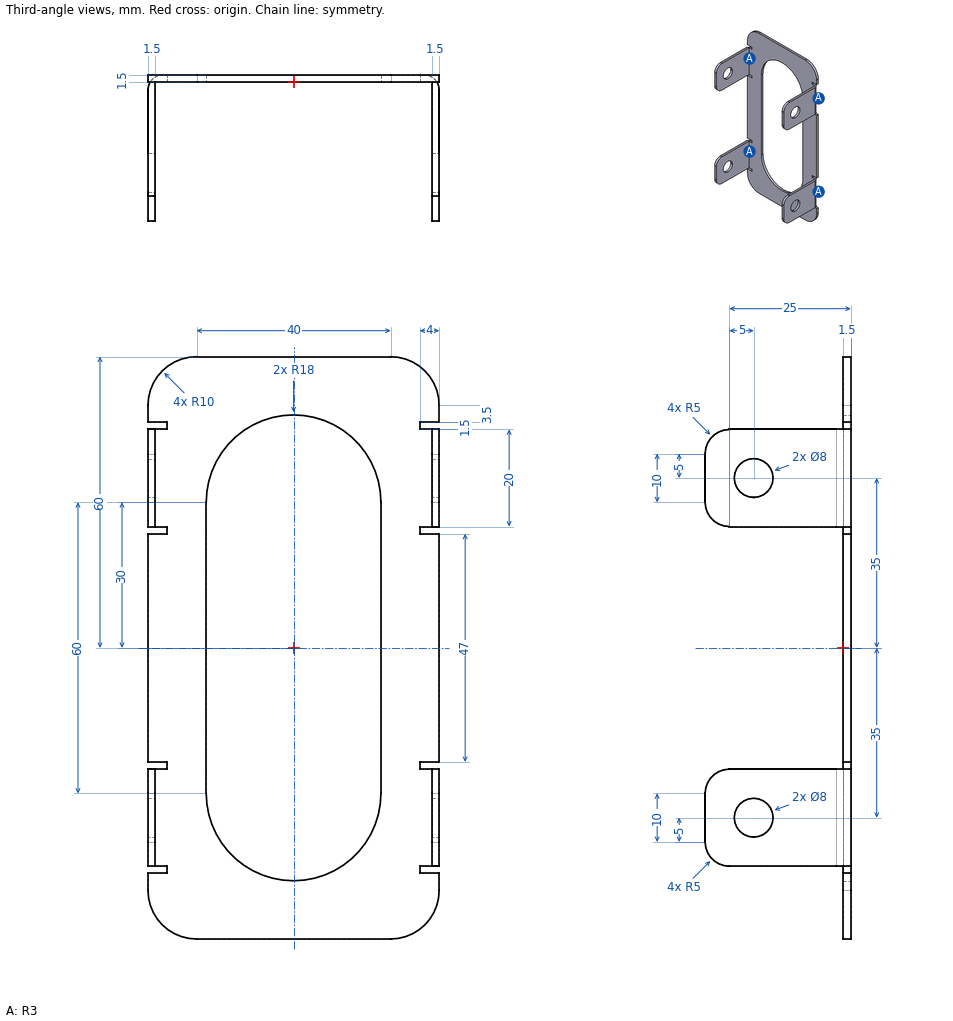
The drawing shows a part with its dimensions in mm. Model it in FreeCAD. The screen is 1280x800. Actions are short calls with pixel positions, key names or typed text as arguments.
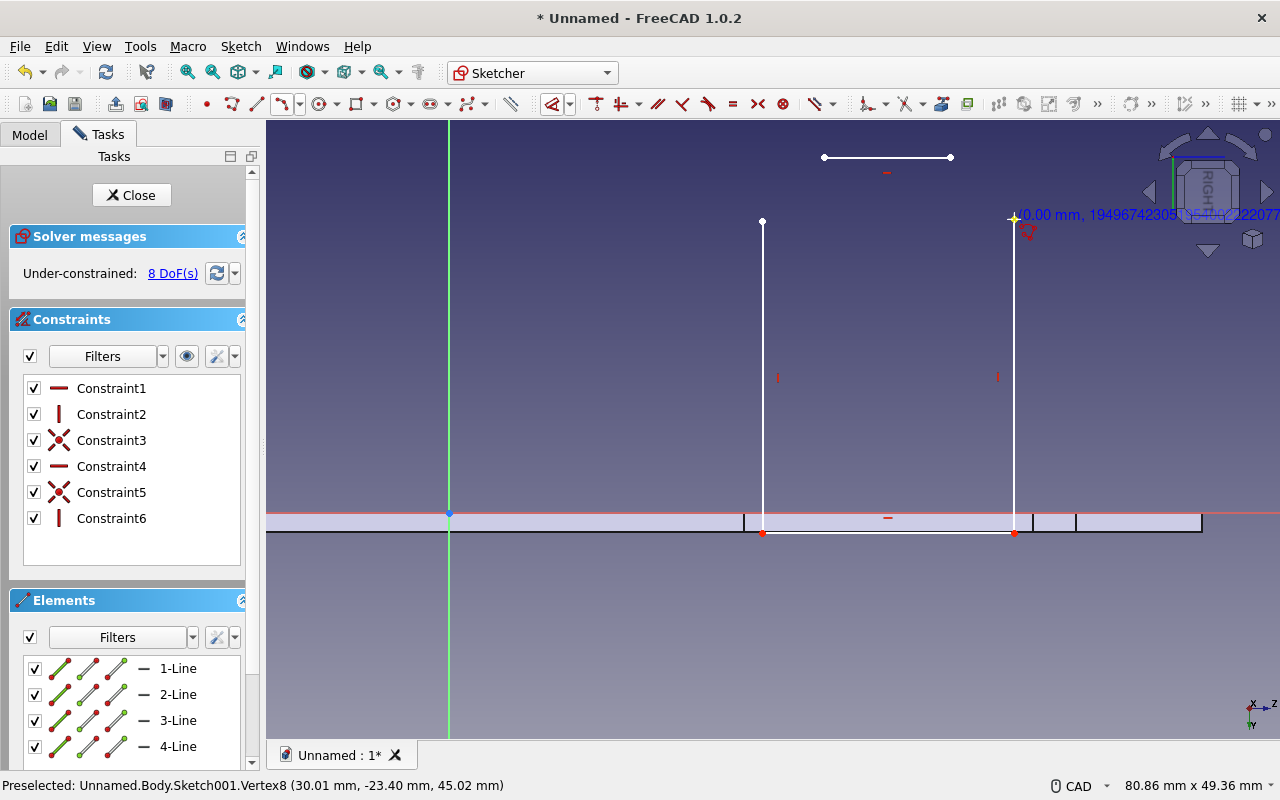
click(282, 104)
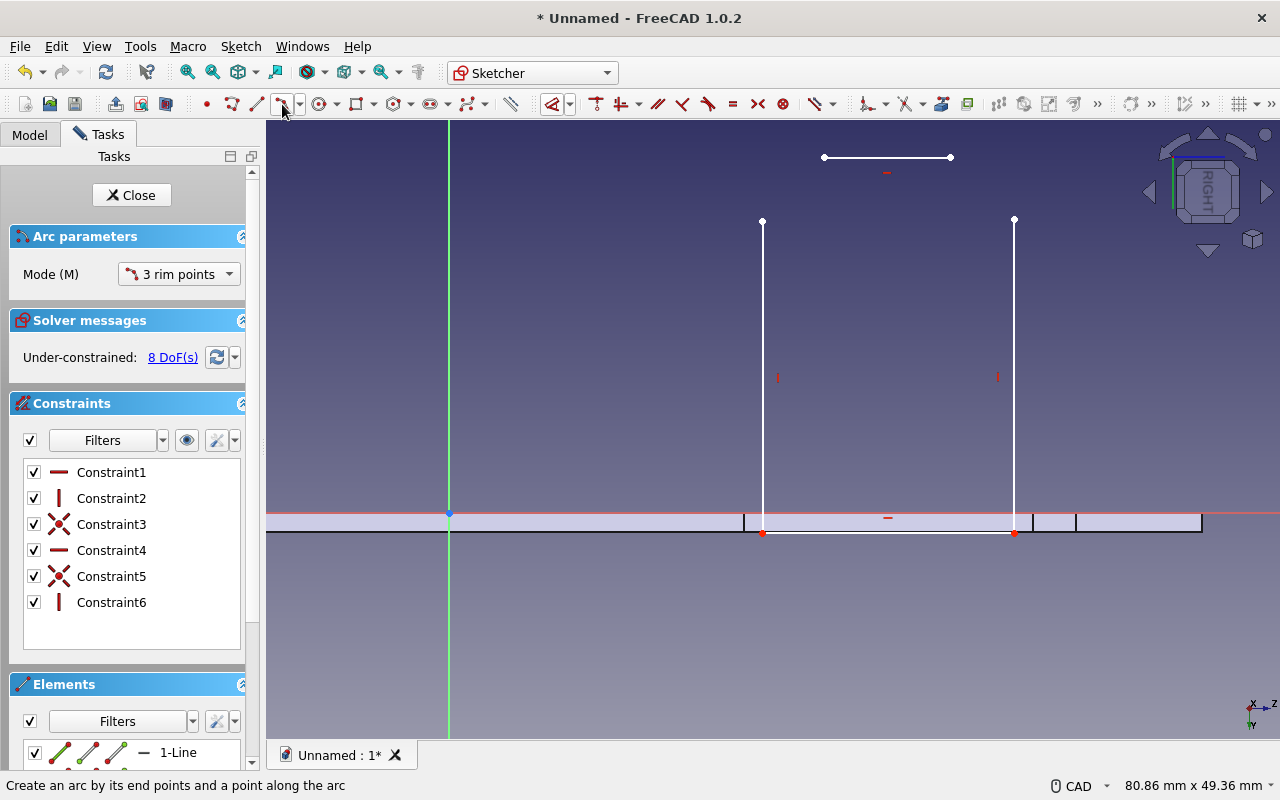
click(825, 158)
click(763, 221)
click(781, 174)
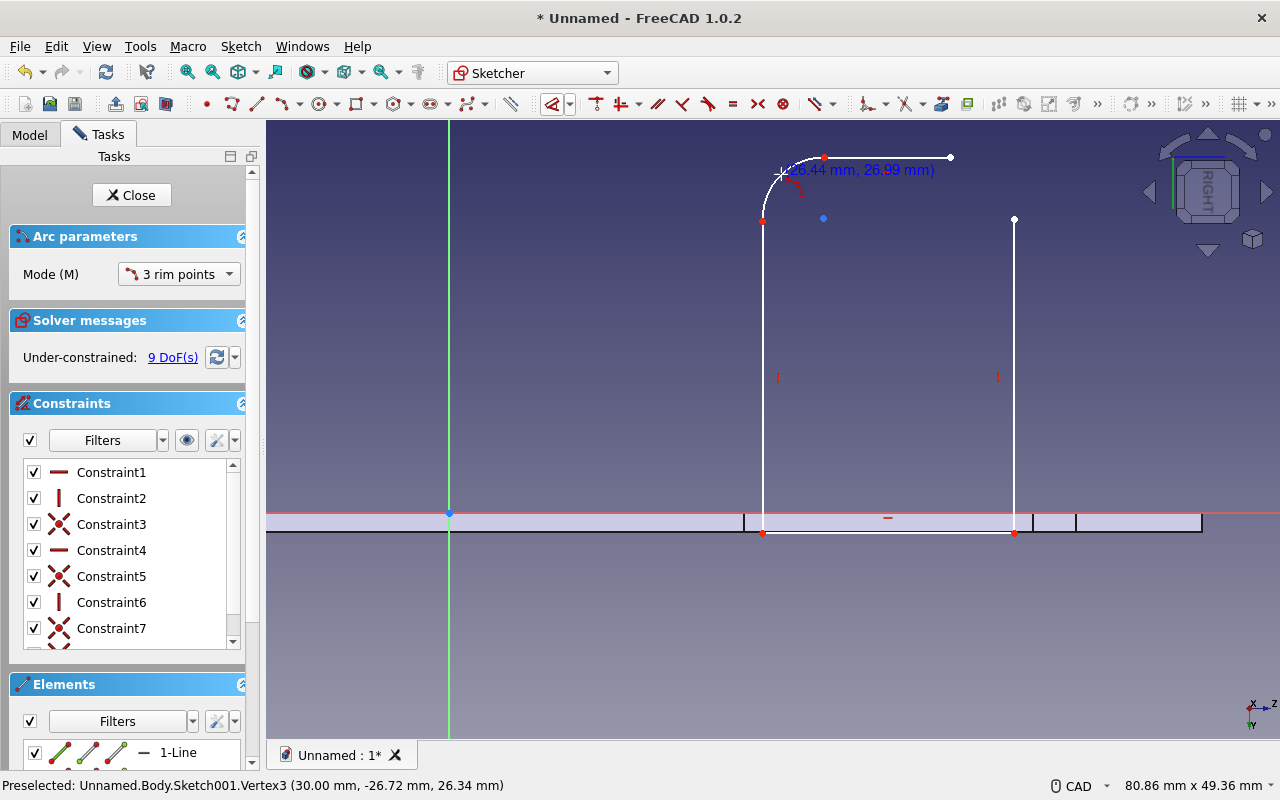
click(1014, 220)
click(951, 158)
click(995, 174)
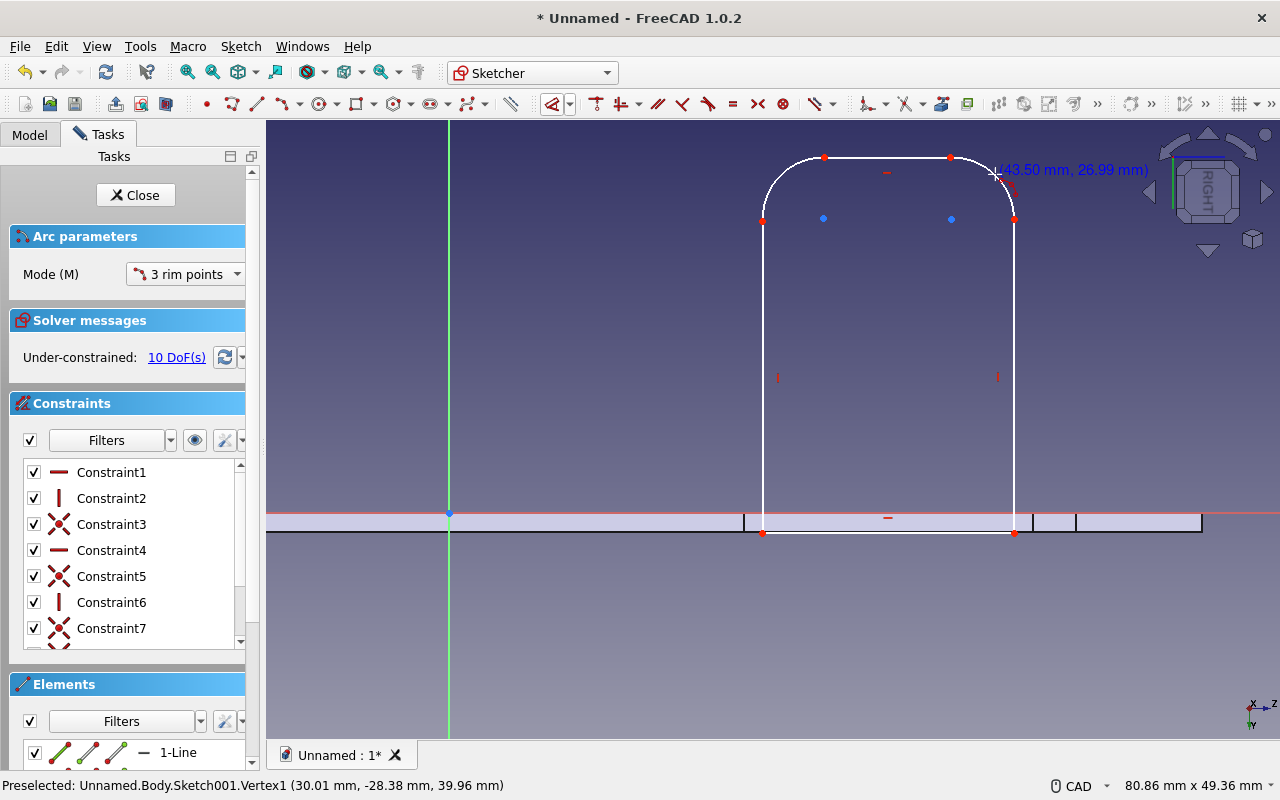
click(257, 104)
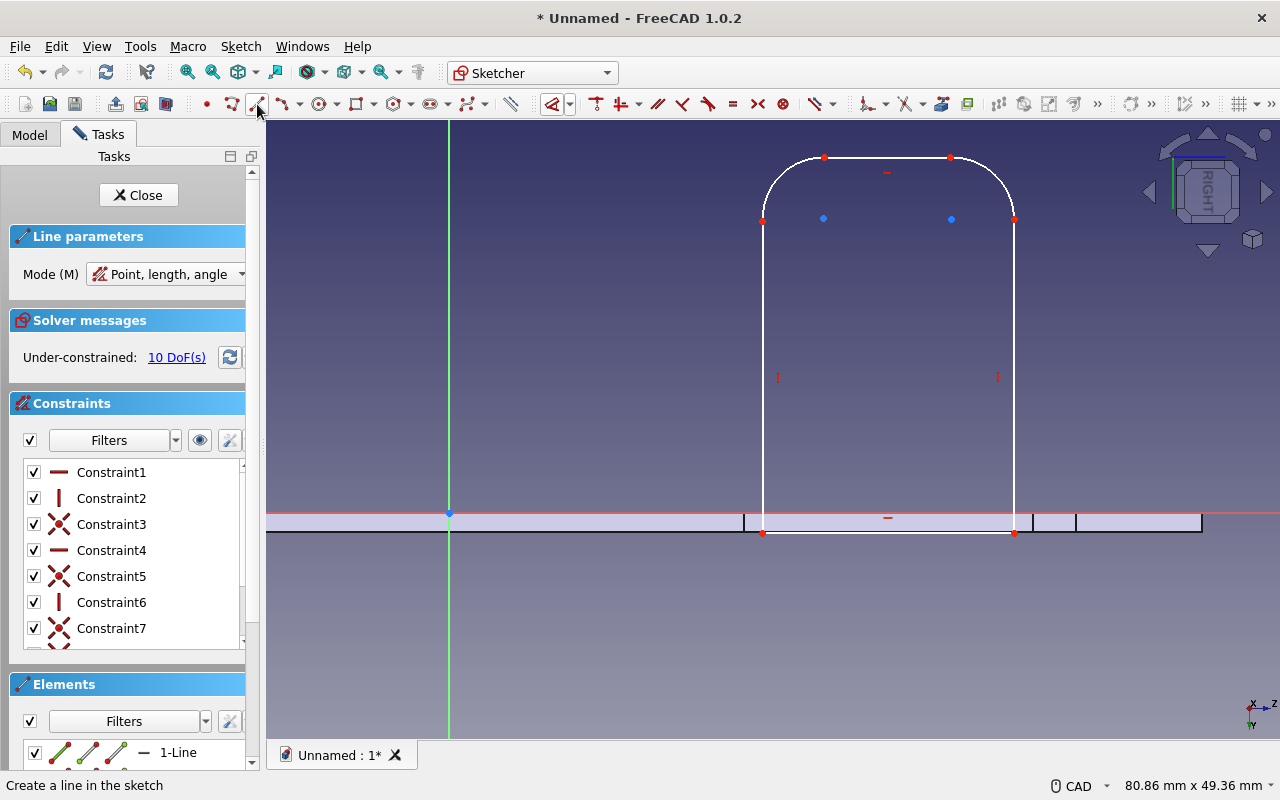
scroll(1015, 533, down, 3)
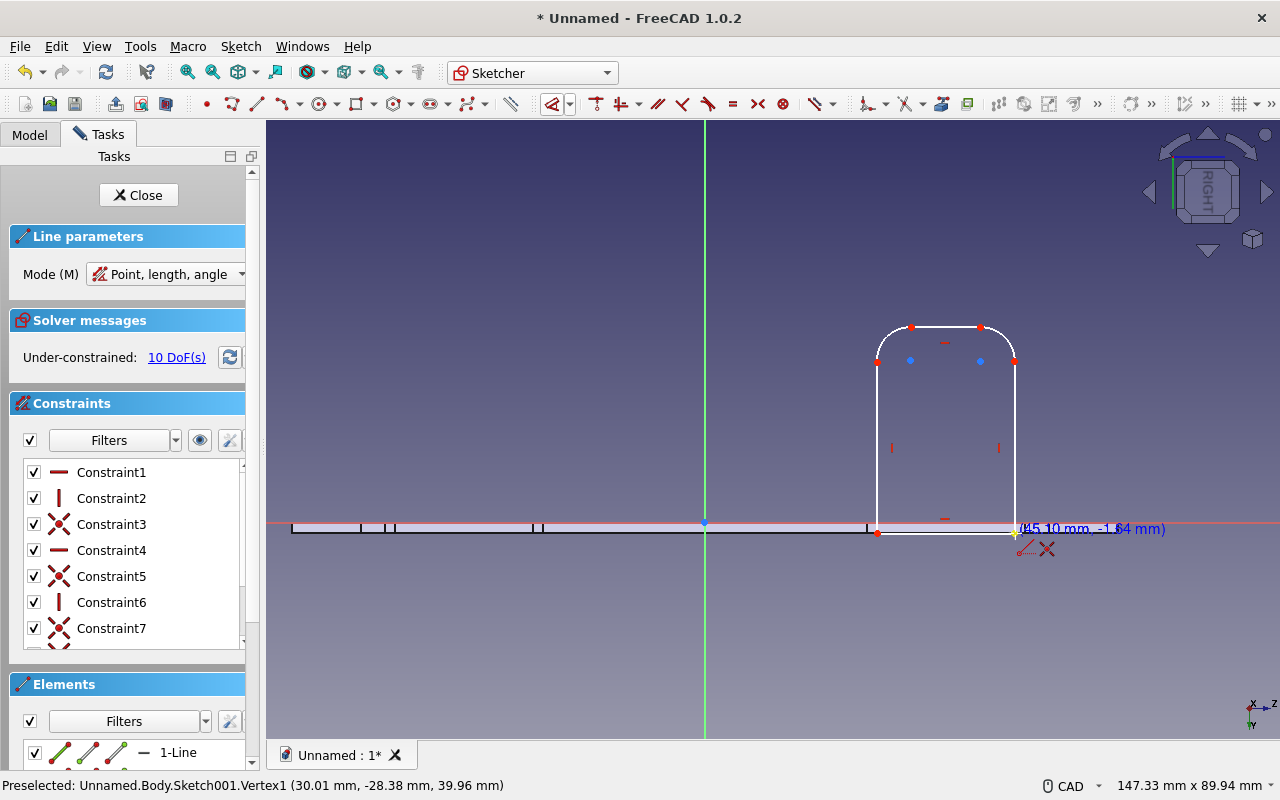
click(498, 326)
click(430, 326)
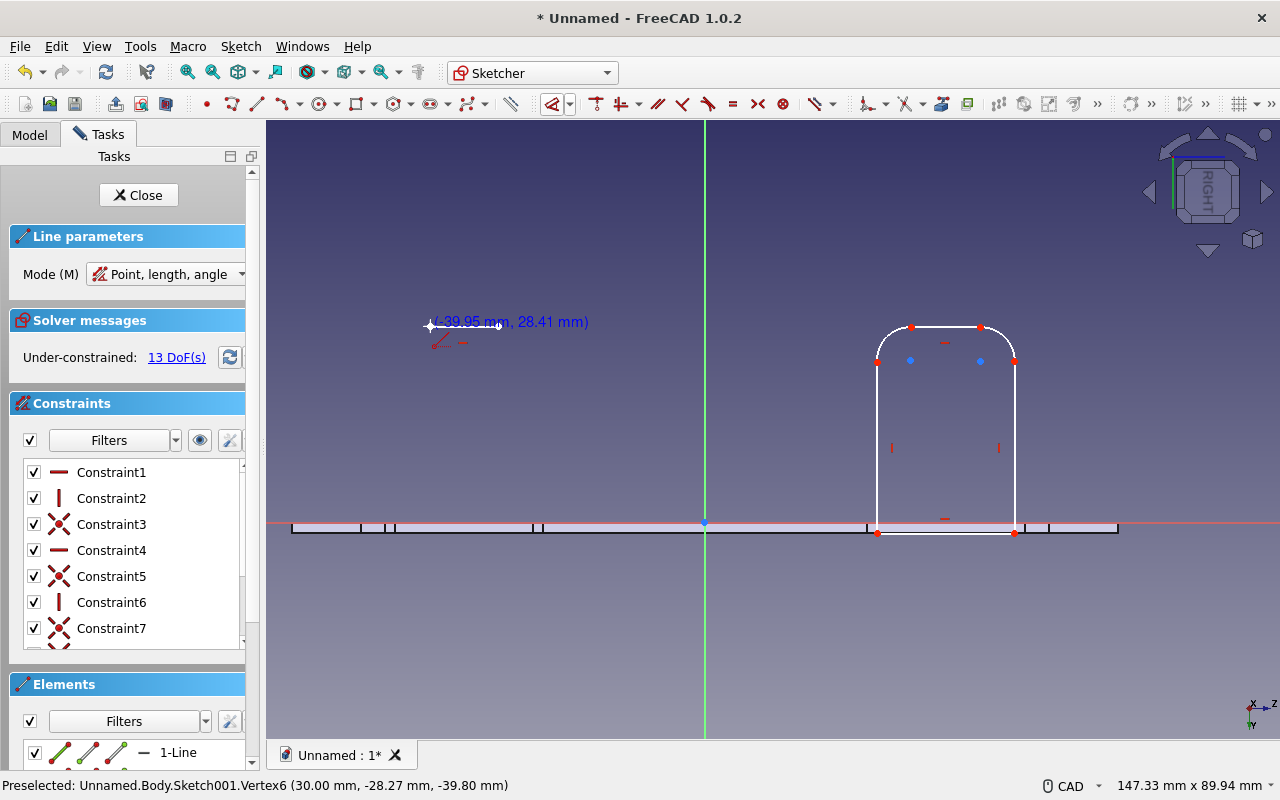
click(232, 104)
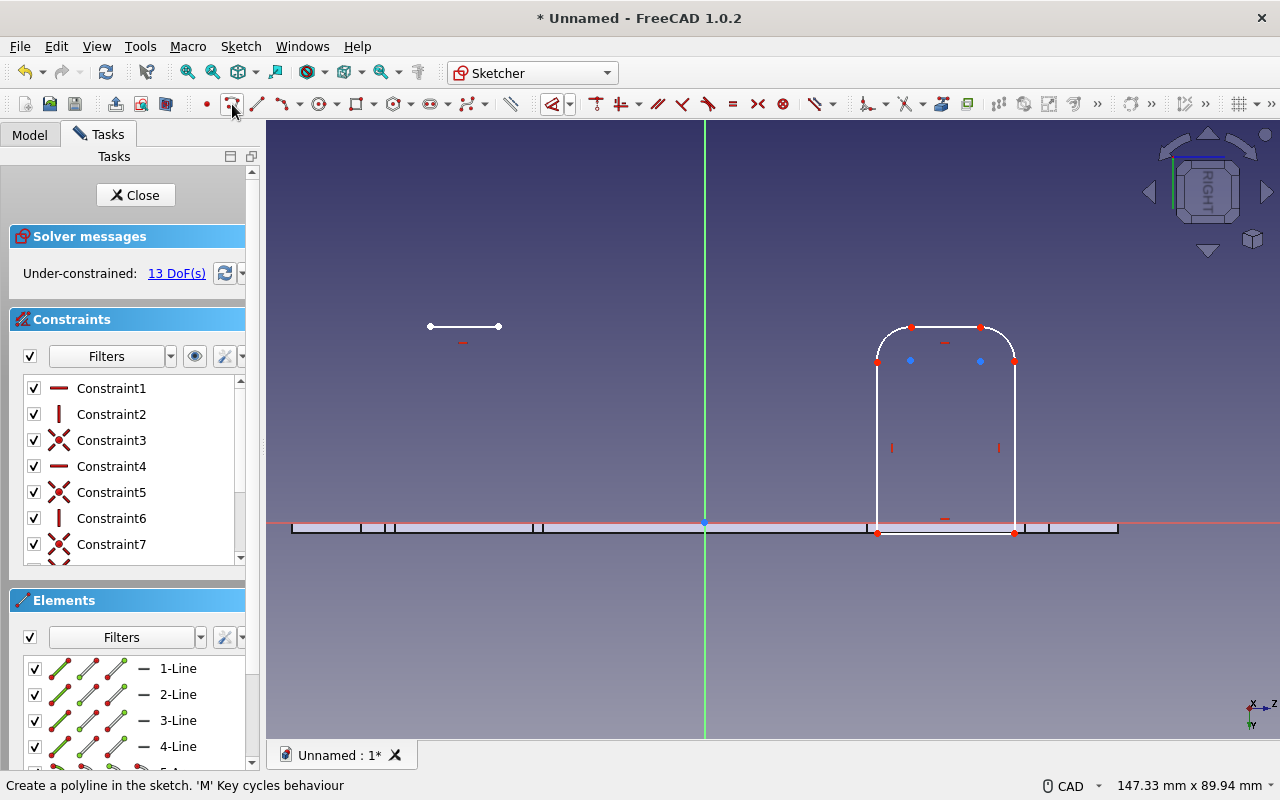
click(395, 361)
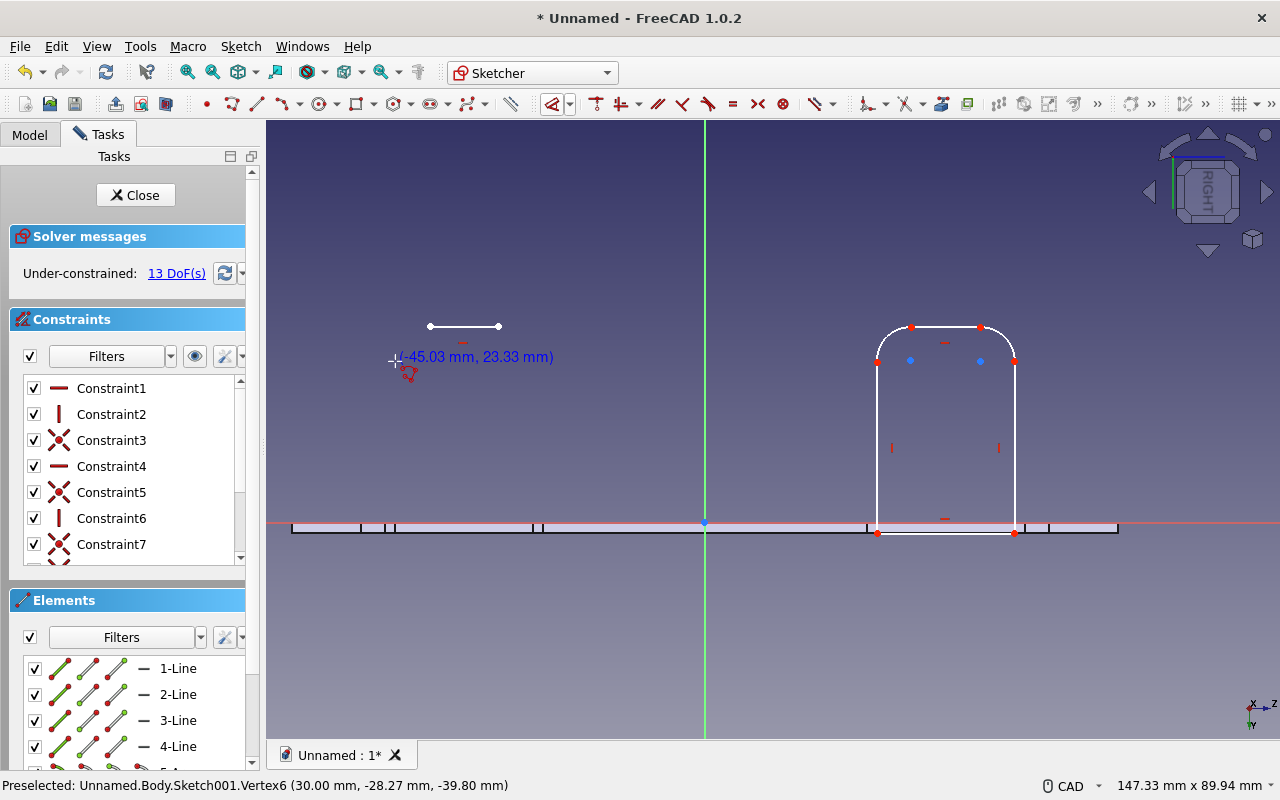
scroll(395, 533, up, 3)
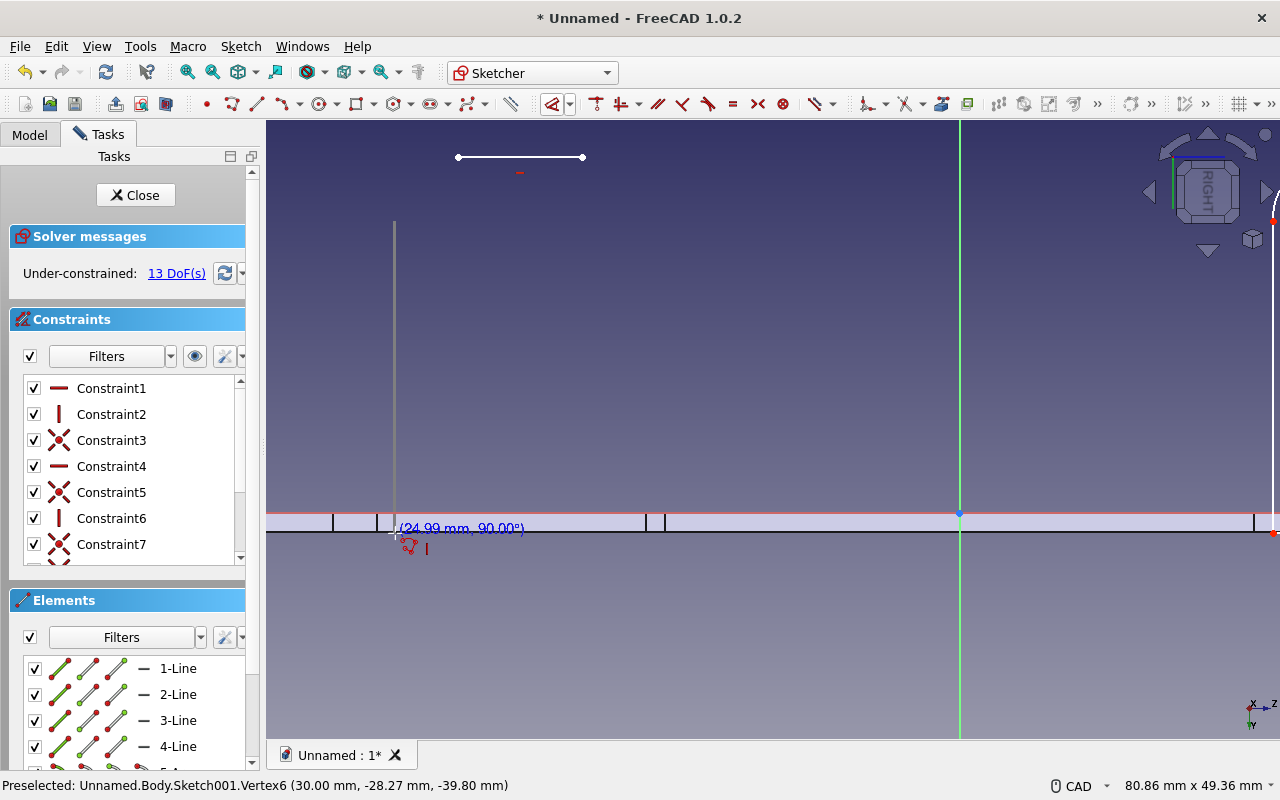
click(395, 532)
click(646, 532)
click(646, 219)
right_click(646, 219)